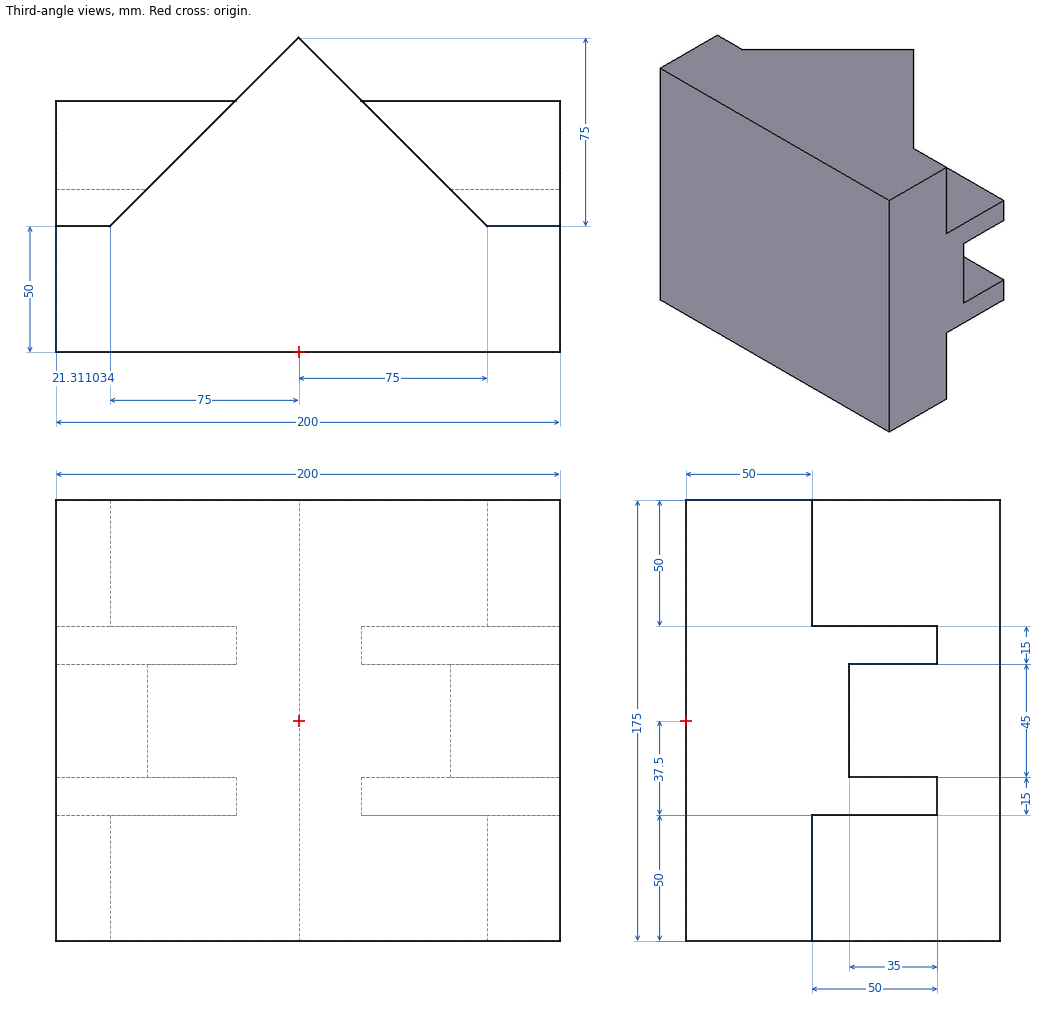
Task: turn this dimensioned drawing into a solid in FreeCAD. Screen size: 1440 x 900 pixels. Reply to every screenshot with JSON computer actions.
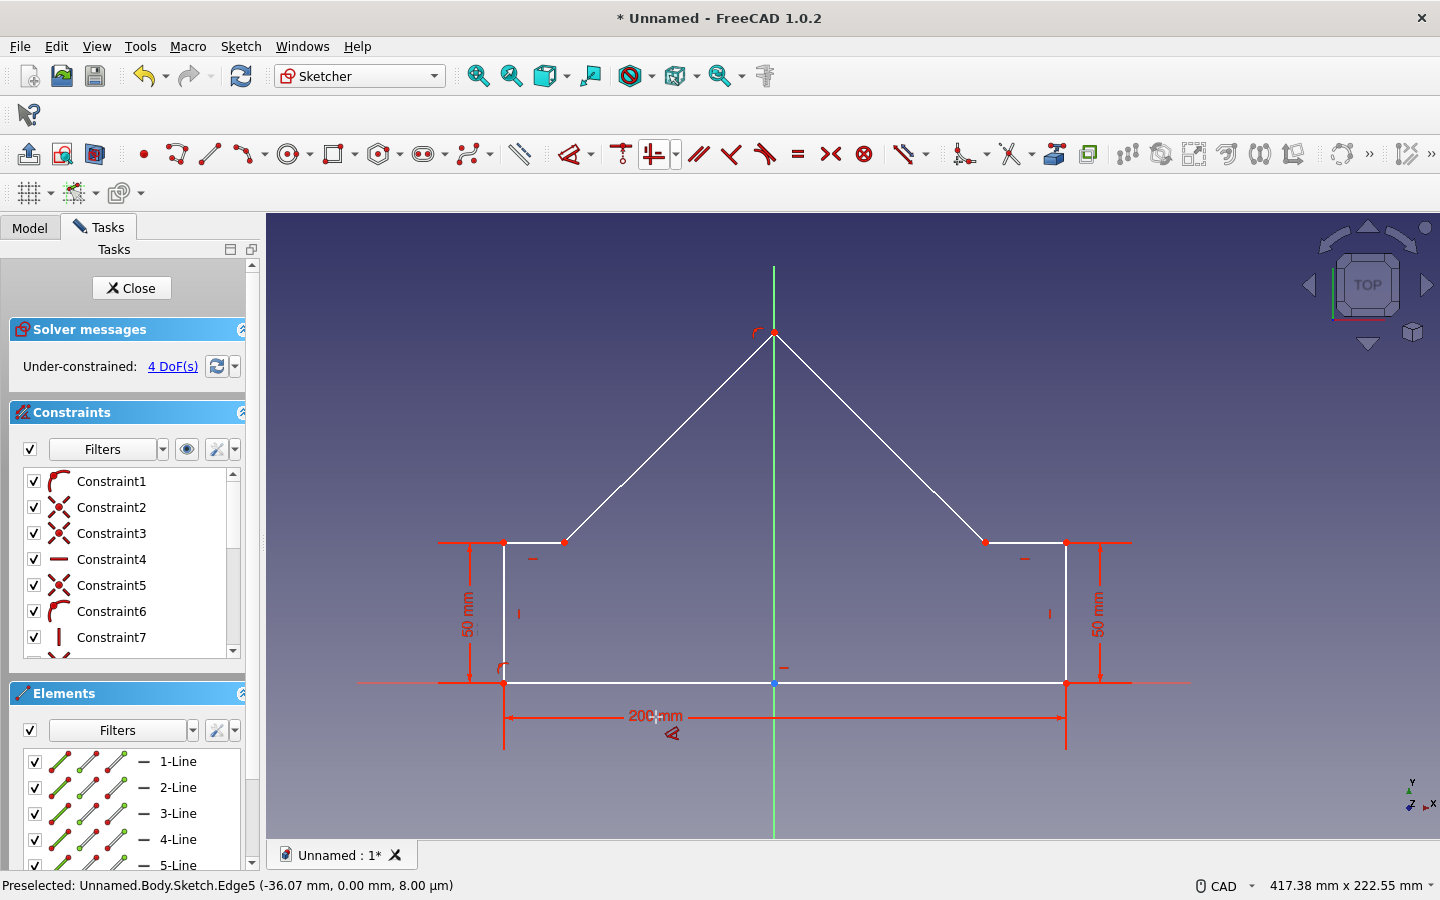
{"action": "left_click", "coordinate": [985, 543]}
{"action": "left_click", "coordinate": [880, 717]}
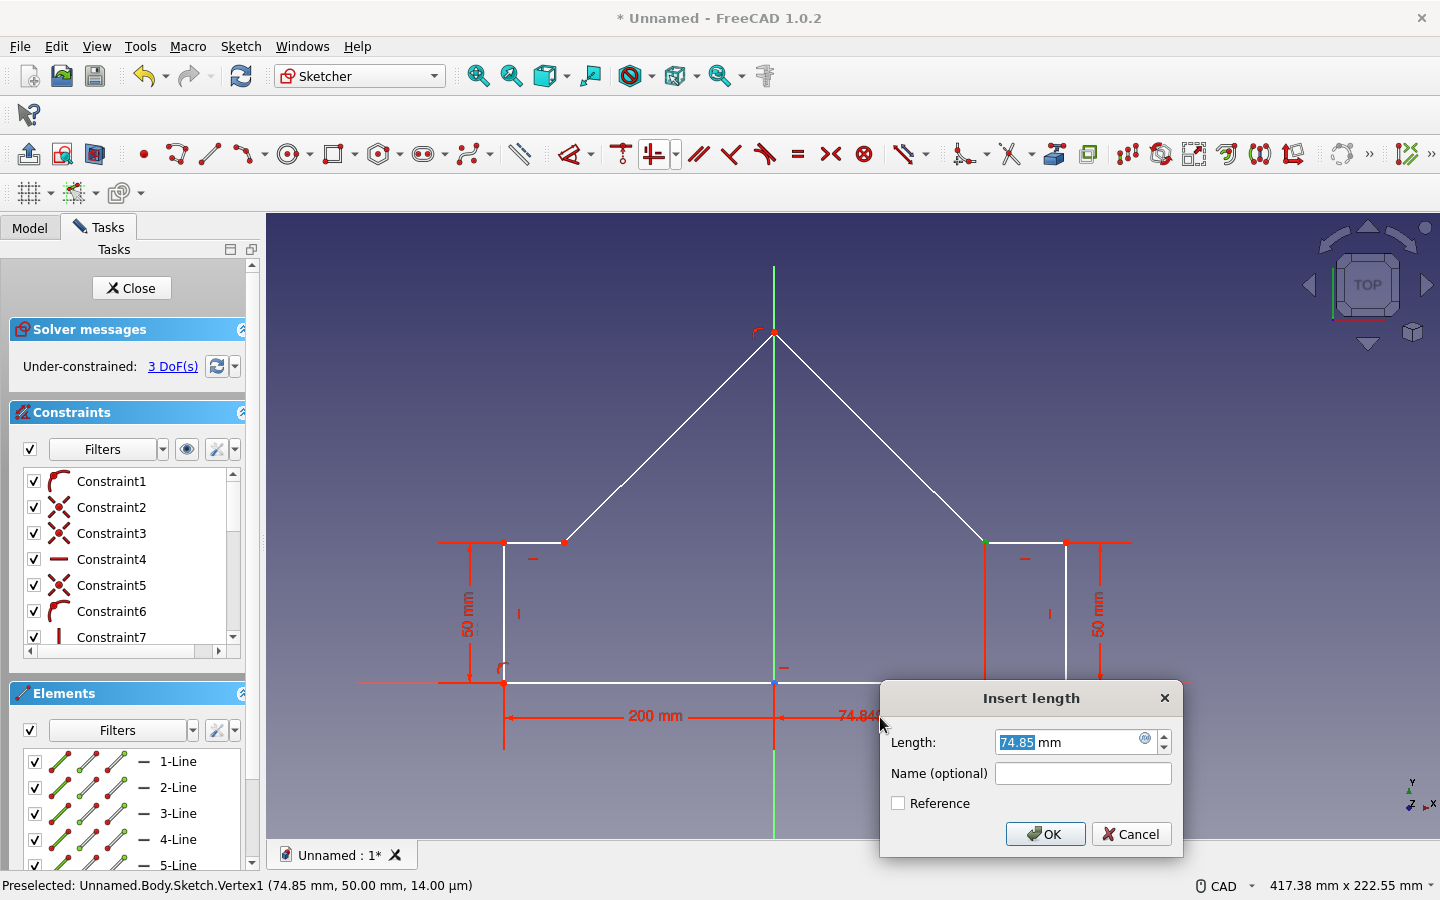
{"action": "type", "text": "75"}
{"action": "key", "text": "Return"}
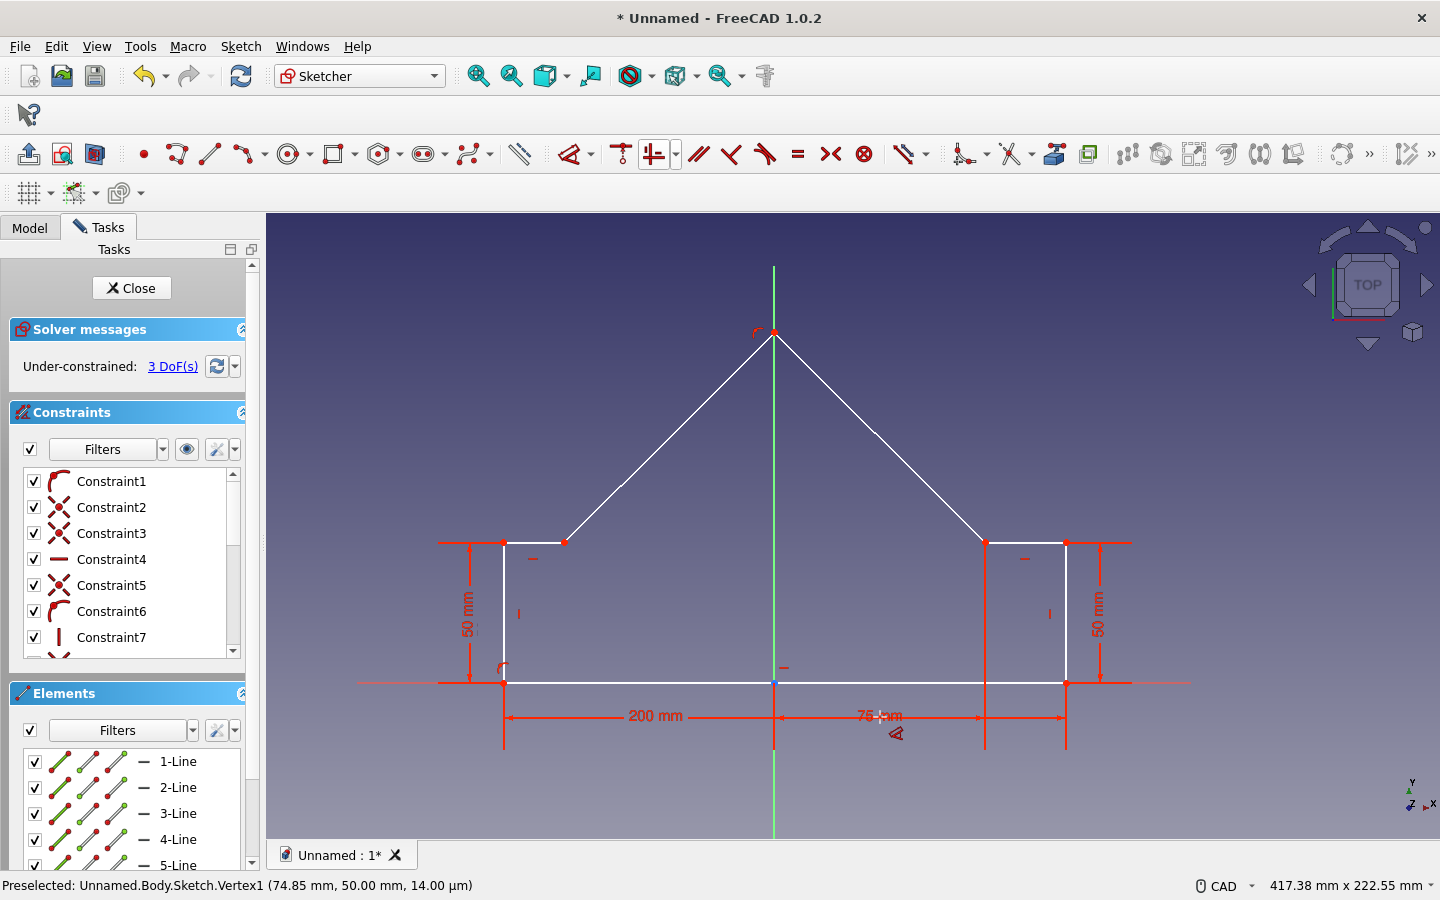
{"action": "left_click", "coordinate": [564, 543]}
{"action": "left_click", "coordinate": [743, 717]}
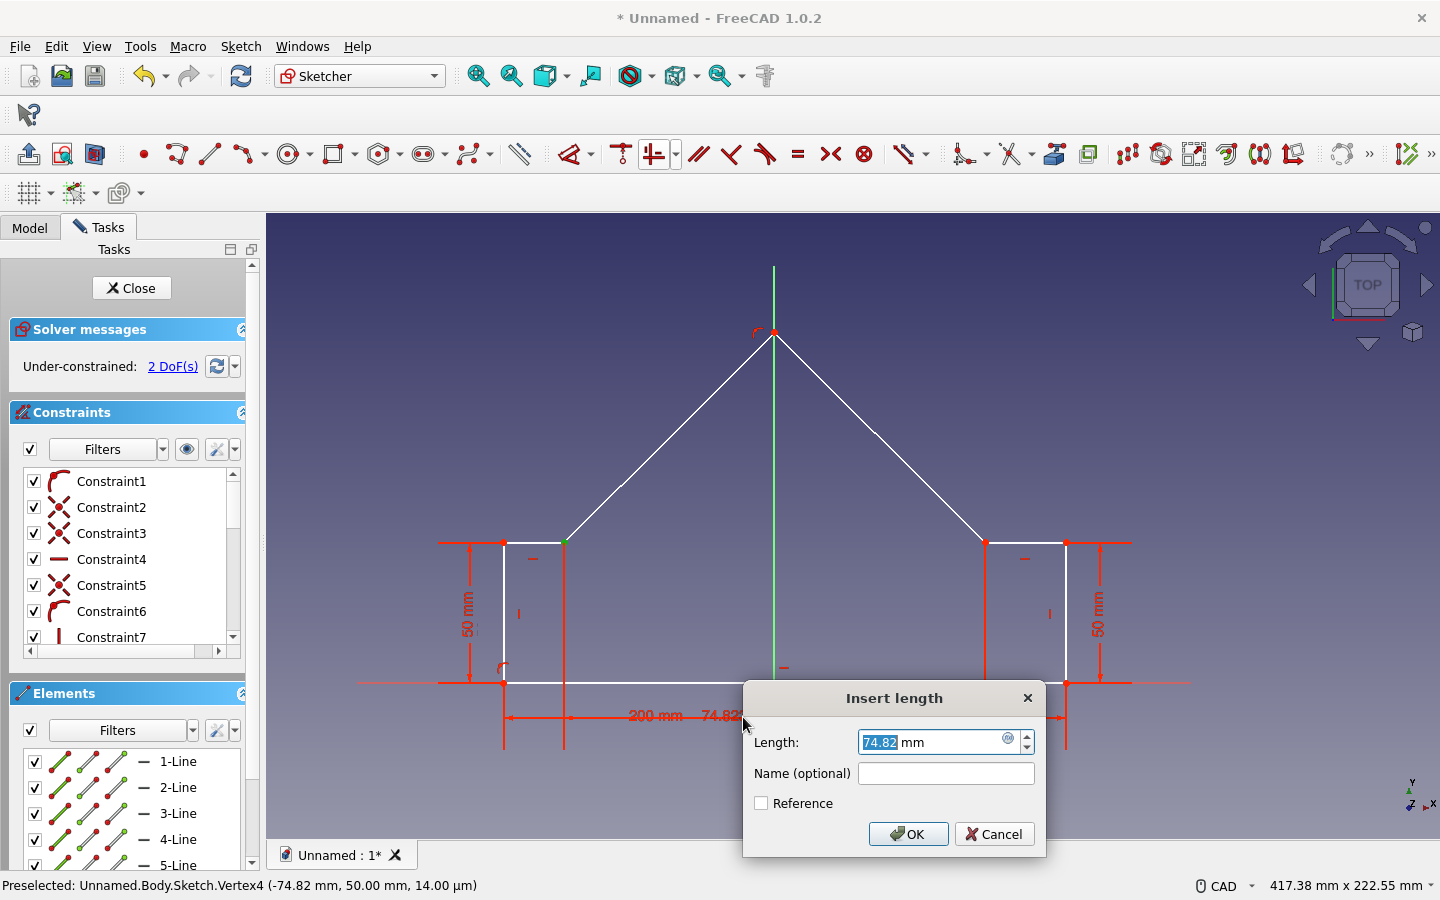
{"action": "type", "text": "75"}
{"action": "key", "text": "Return"}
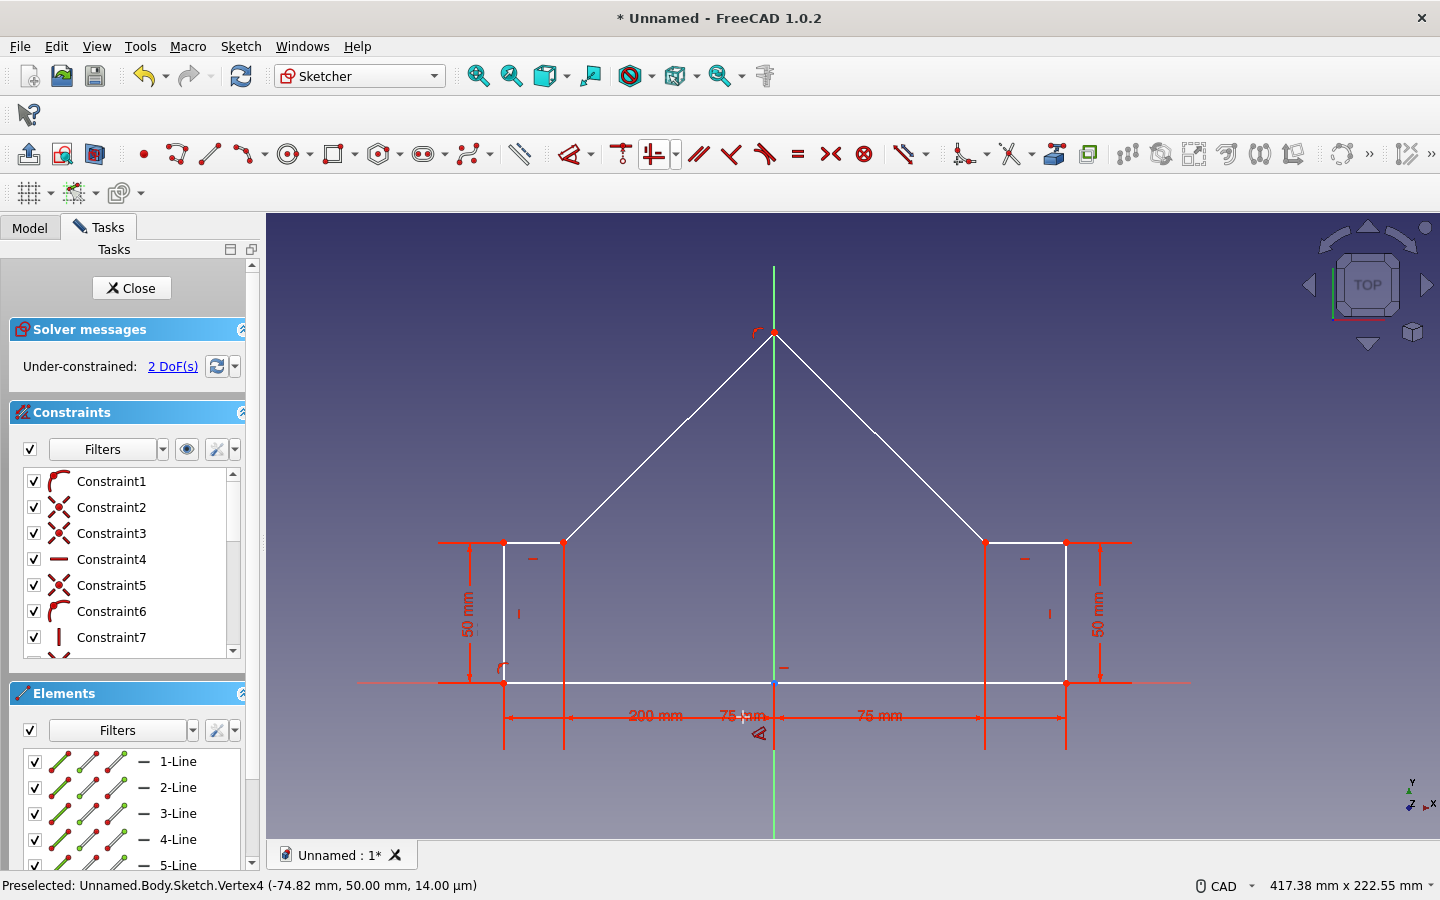
{"action": "left_click", "coordinate": [922, 480]}
{"action": "left_click", "coordinate": [1019, 438]}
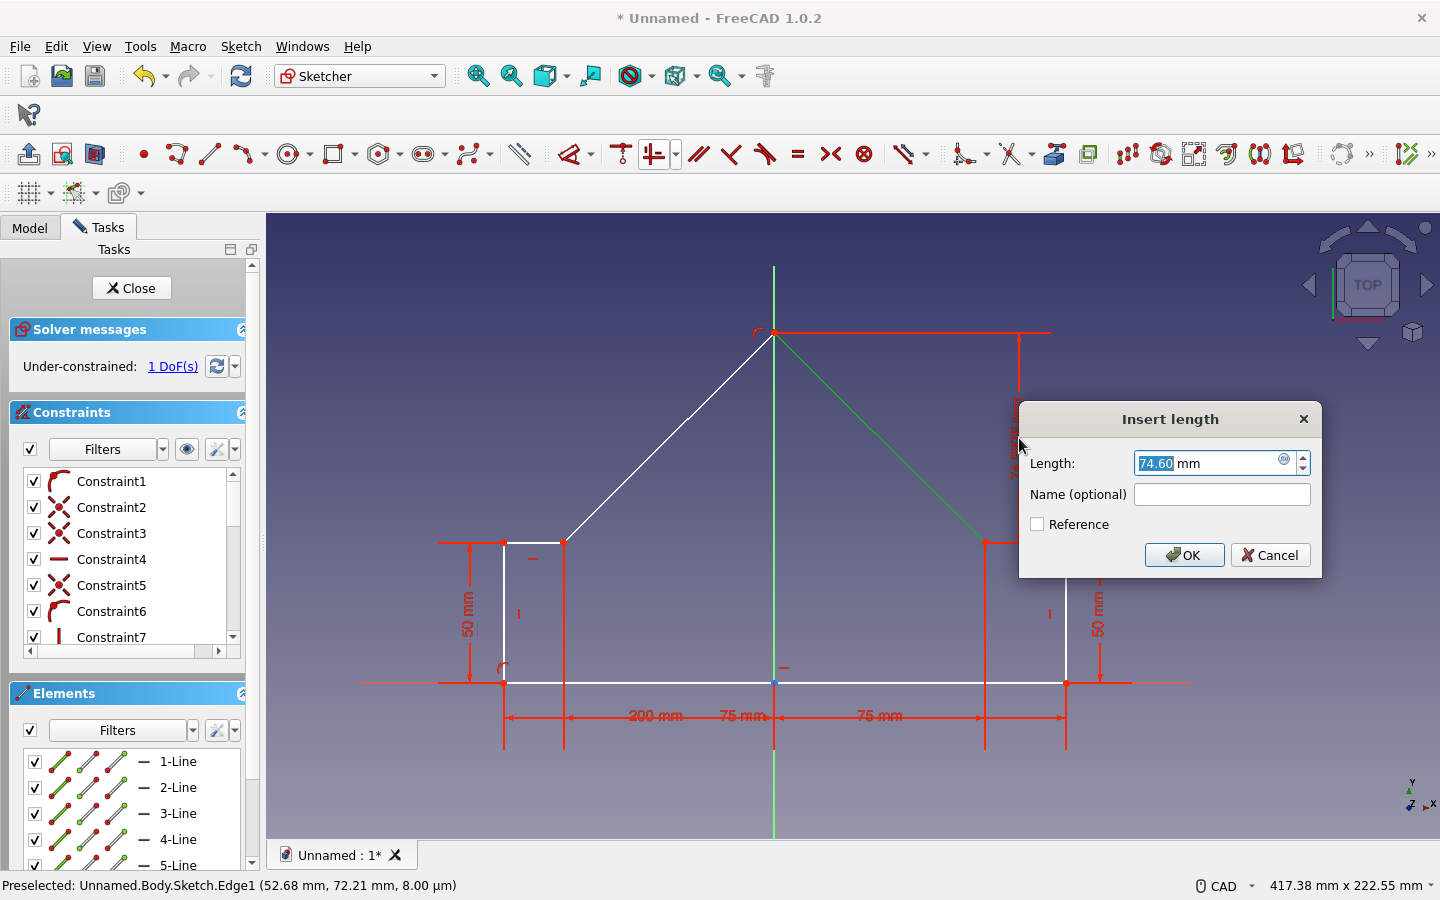
{"action": "type", "text": "75"}
{"action": "key", "text": "Return"}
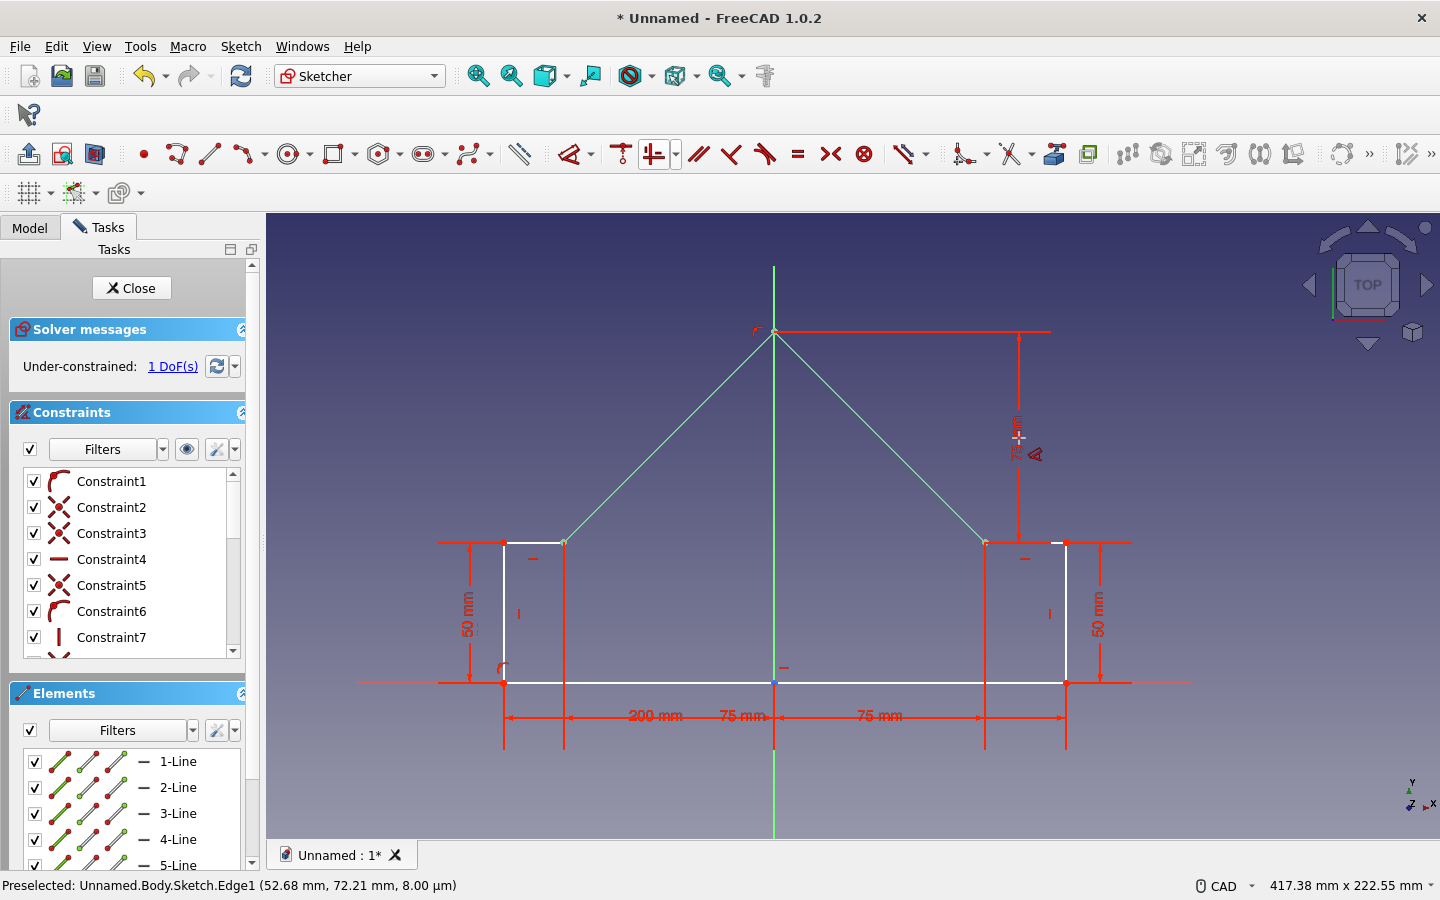
{"action": "left_click", "coordinate": [546, 543]}
{"action": "left_click", "coordinate": [534, 577]}